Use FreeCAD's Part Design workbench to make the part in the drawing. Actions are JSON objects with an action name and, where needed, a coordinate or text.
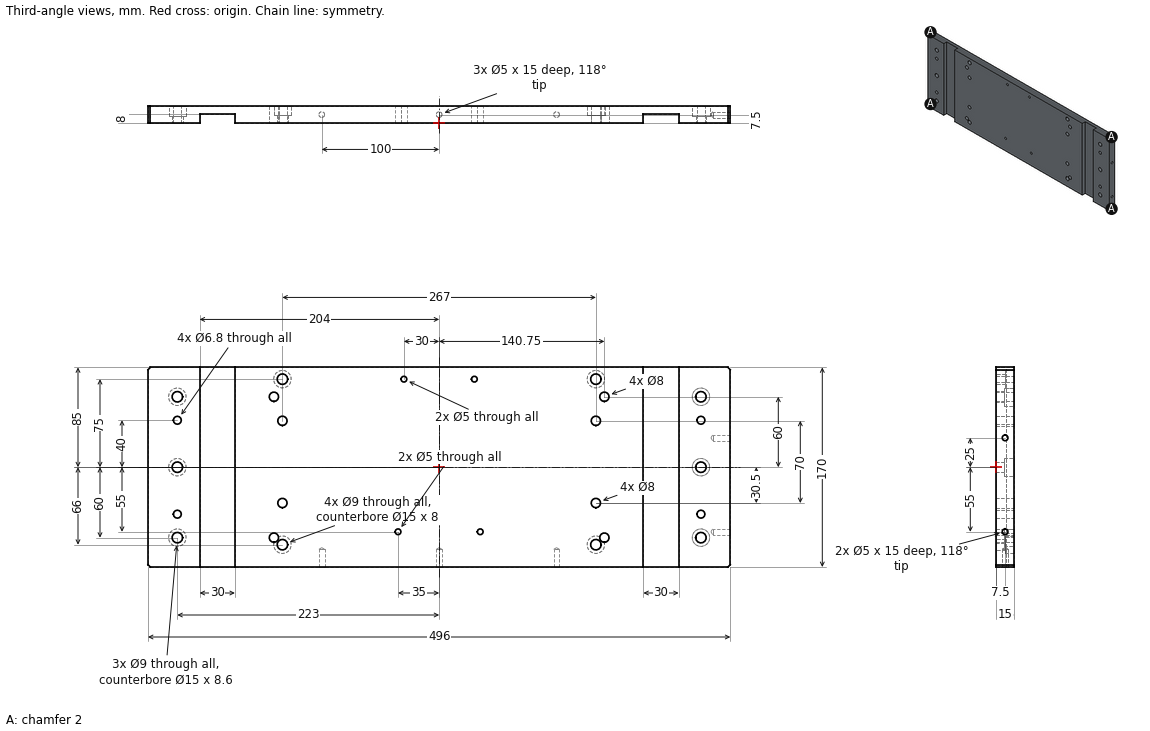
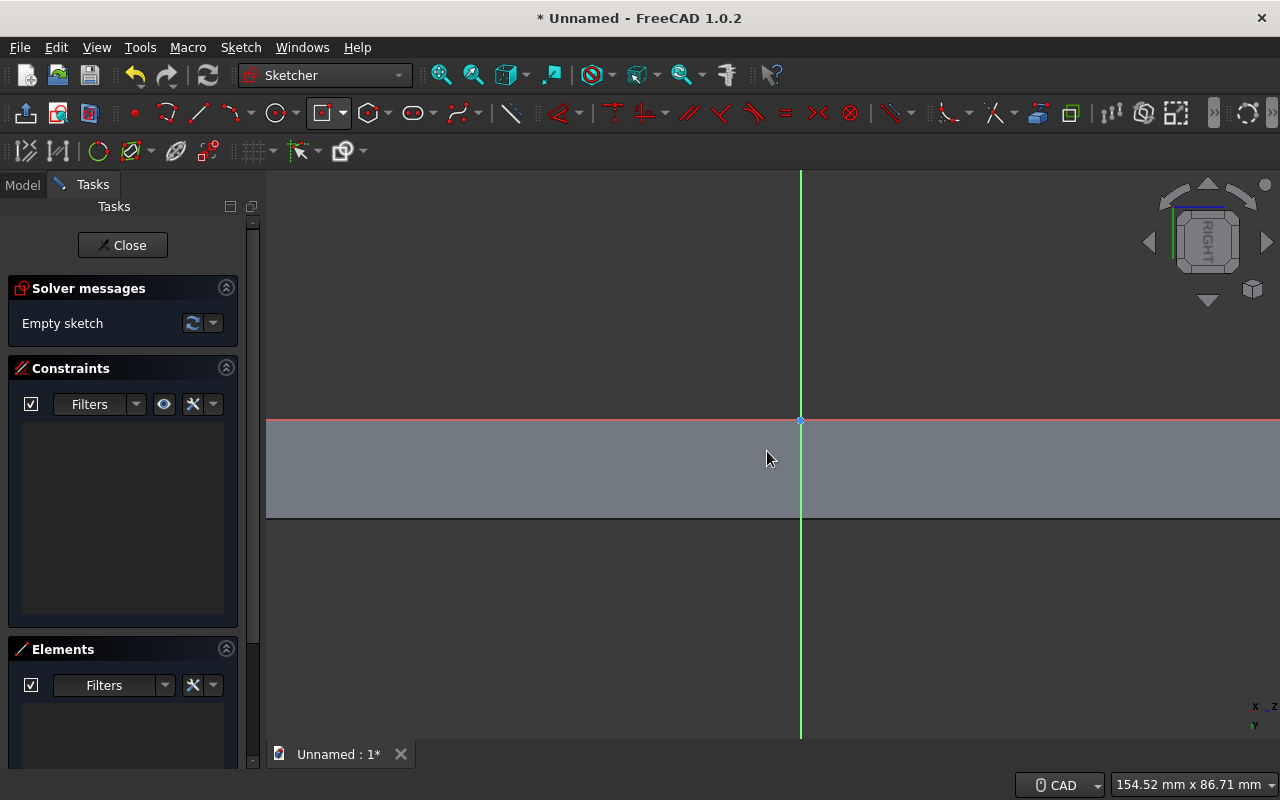
{"action": "left_click", "coordinate": [276, 114]}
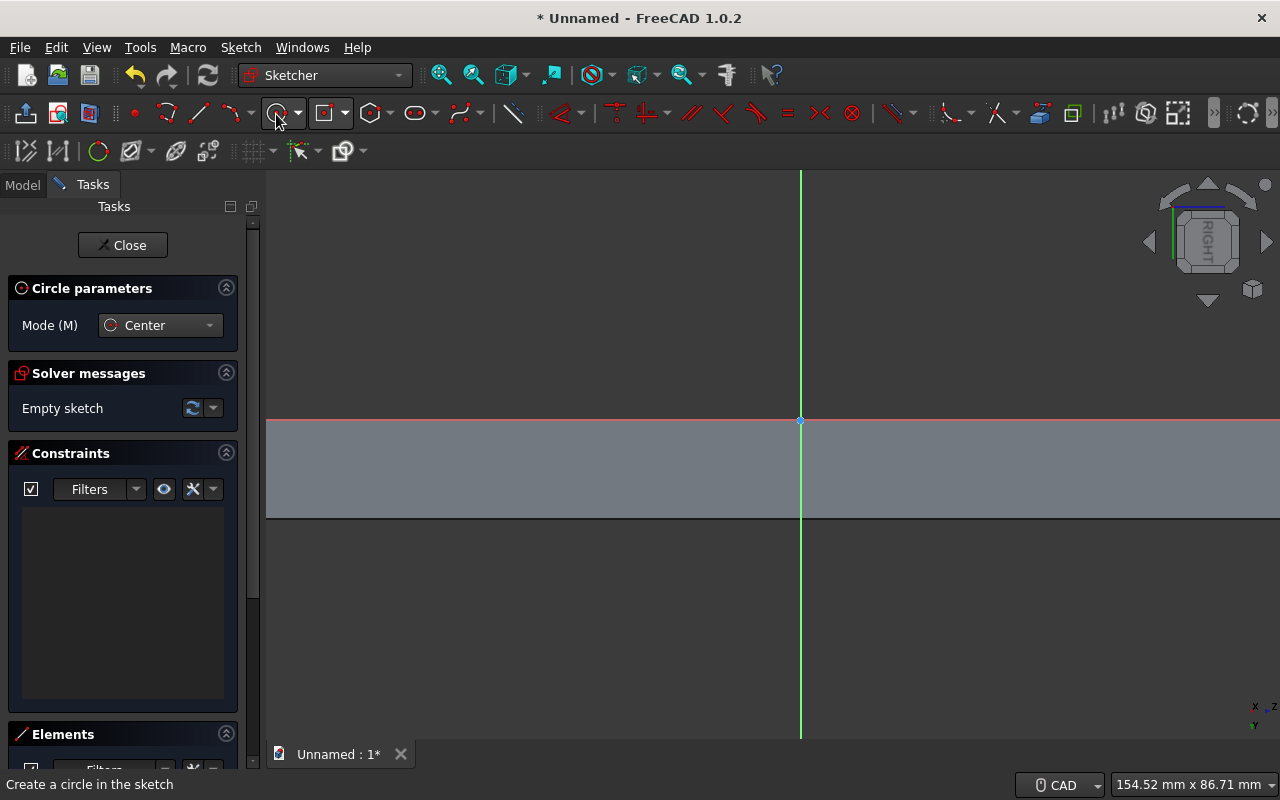
{"action": "scroll", "coordinate": [440, 470], "scroll_direction": "up", "scroll_amount": 2}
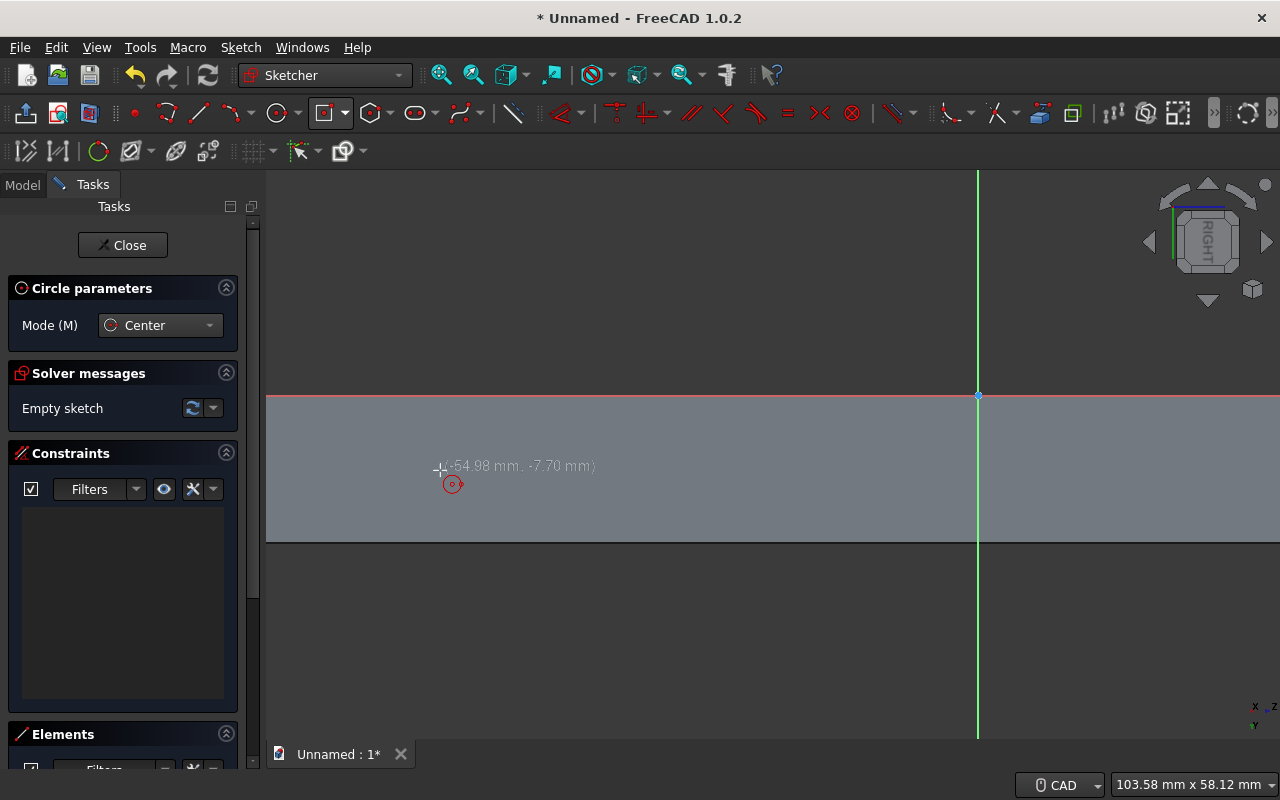
{"action": "left_click", "coordinate": [440, 469]}
{"action": "mouse_move", "coordinate": [457, 452]}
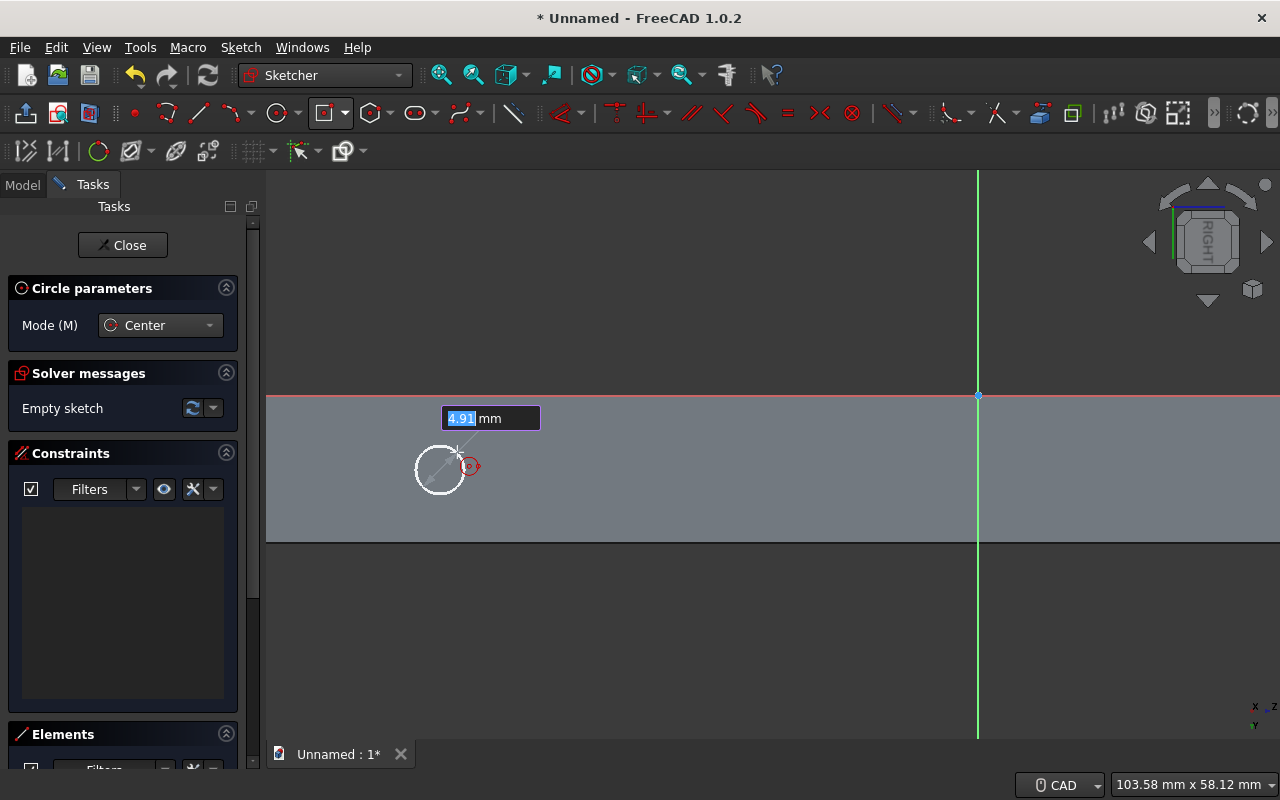
{"action": "type", "text": "5"}
{"action": "key", "text": "Return"}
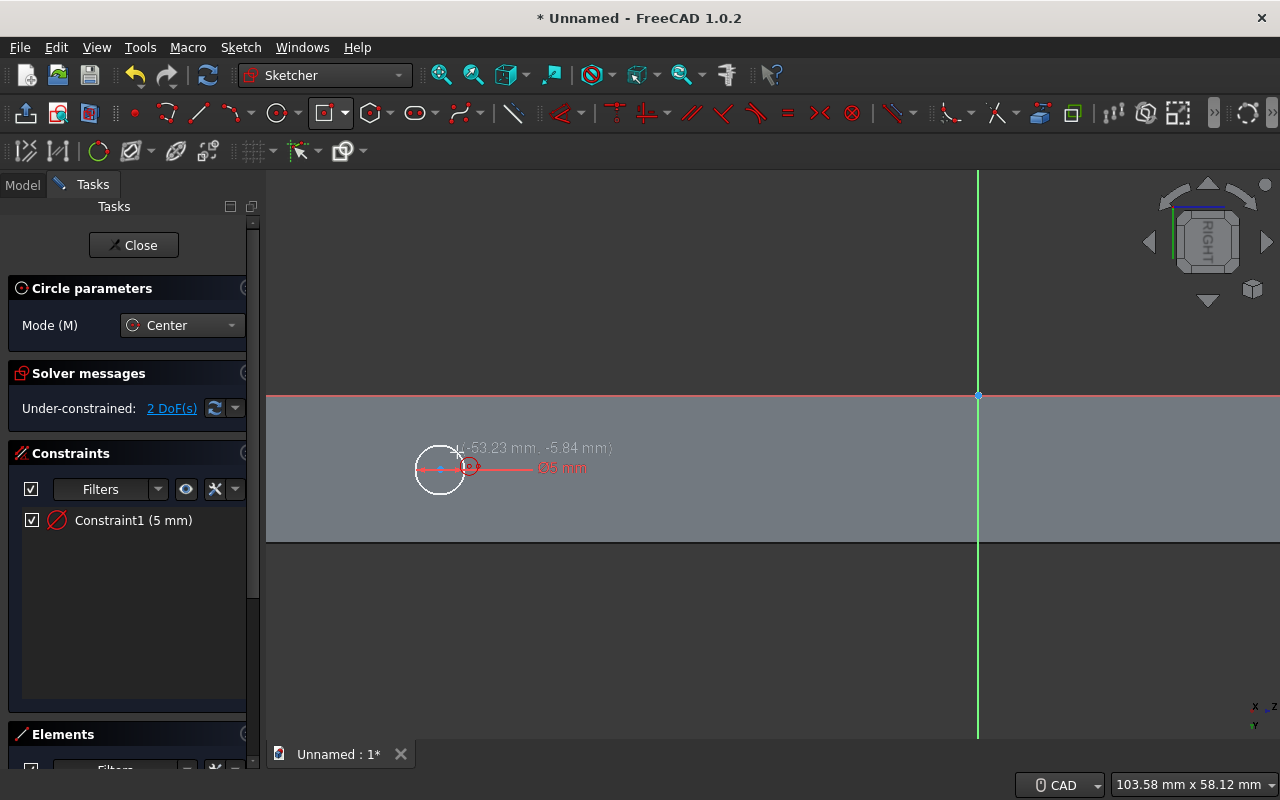
{"action": "scroll", "coordinate": [447, 474], "scroll_direction": "down", "scroll_amount": 2}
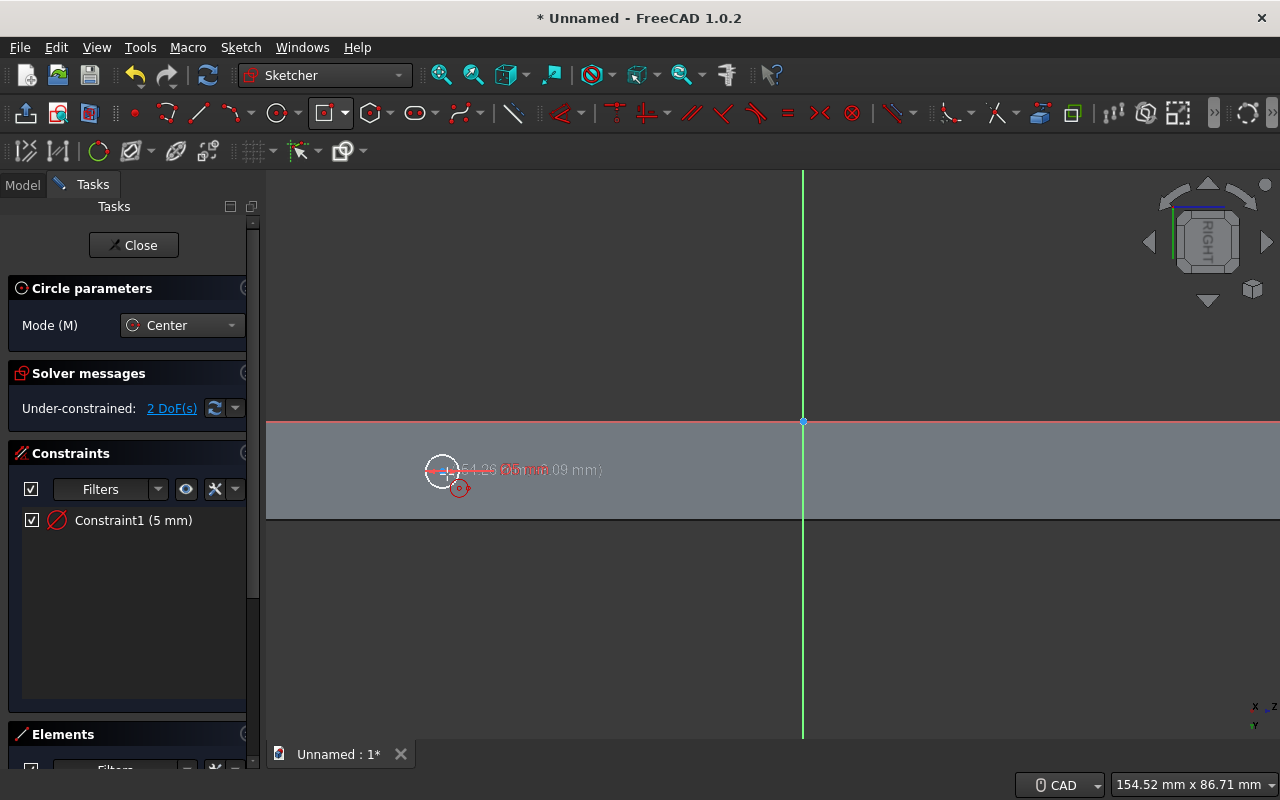
{"action": "scroll", "coordinate": [967, 471], "scroll_direction": "up", "scroll_amount": 2}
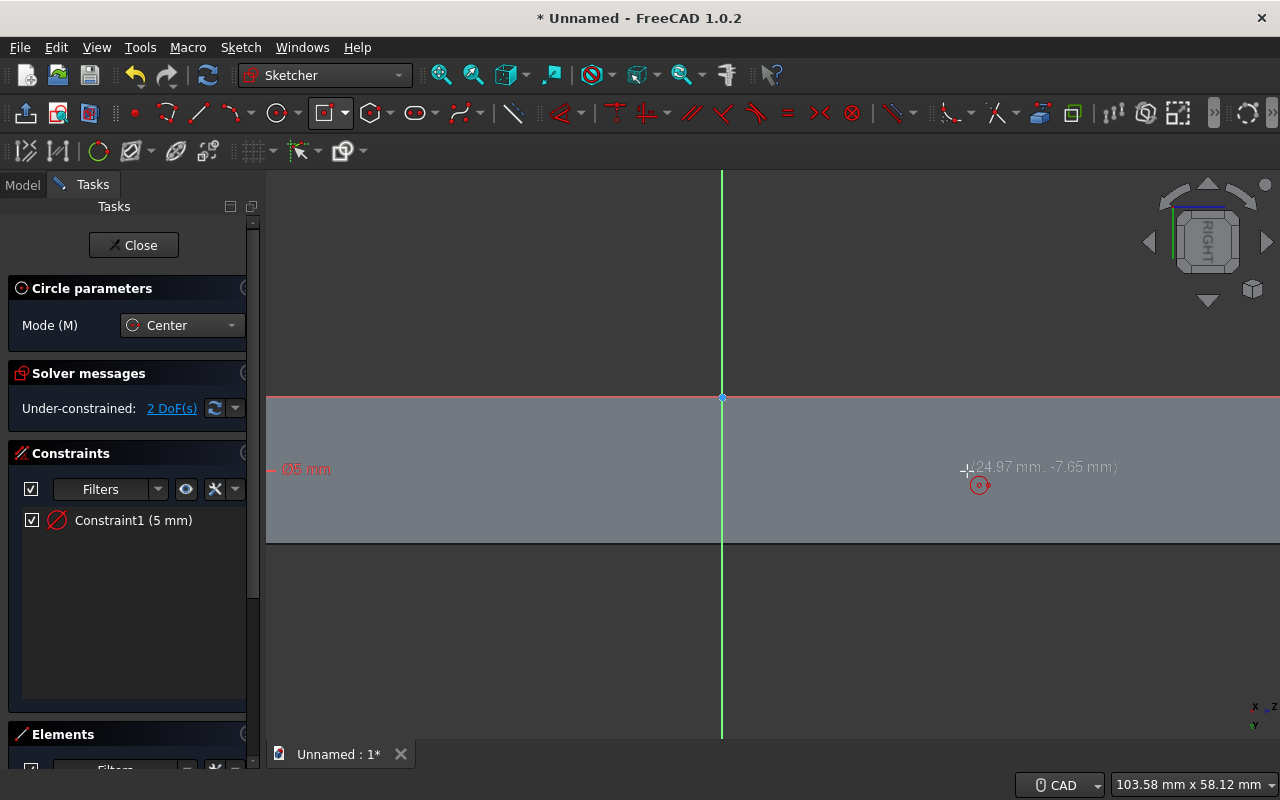
{"action": "left_click", "coordinate": [967, 471]}
{"action": "mouse_move", "coordinate": [984, 453]}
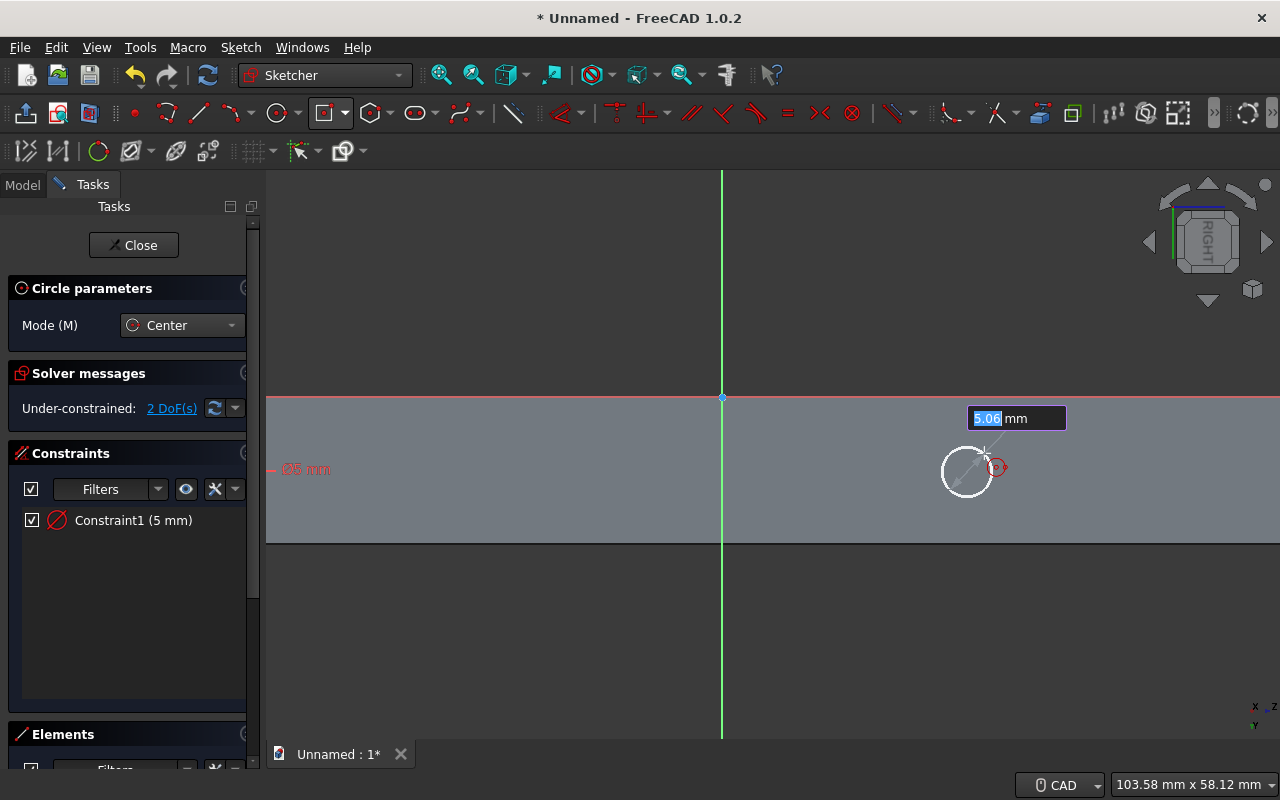
{"action": "type", "text": "5"}
{"action": "key", "text": "Return"}
{"action": "key", "text": "Escape"}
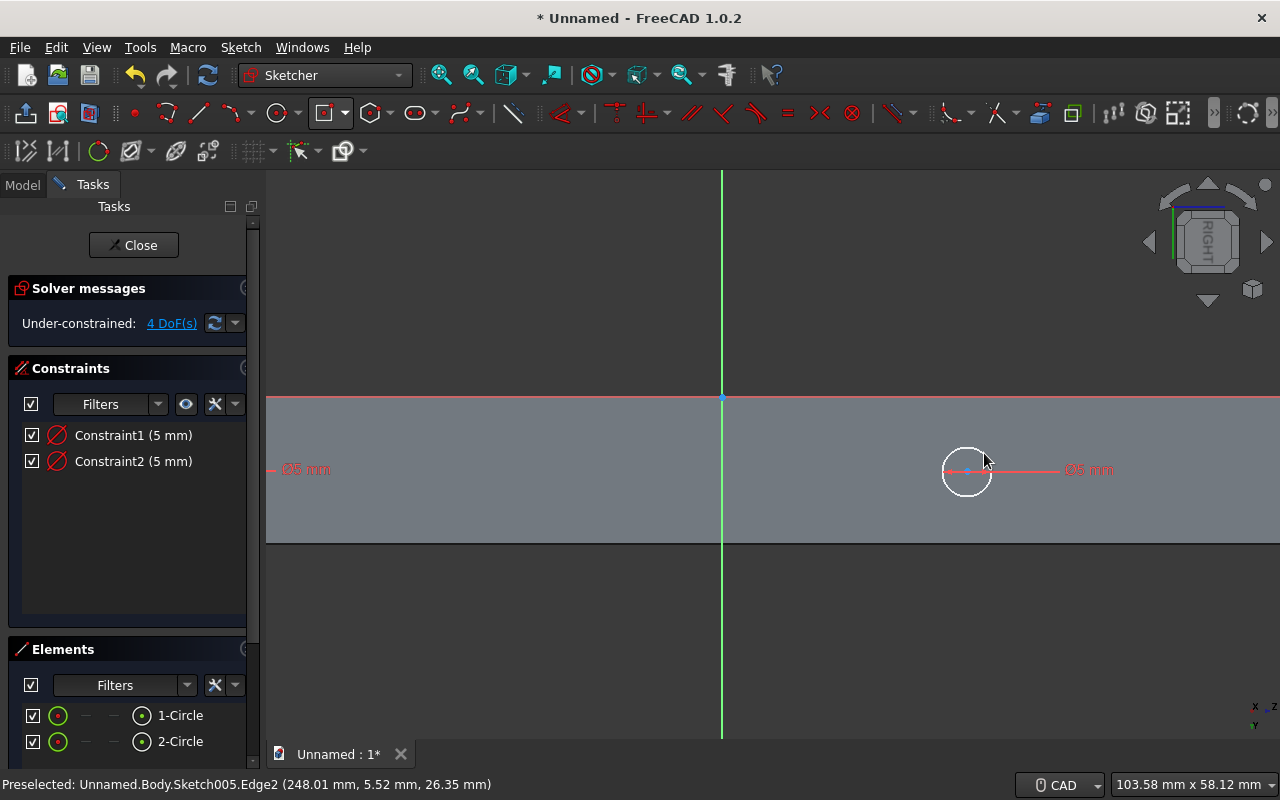
{"action": "left_click", "coordinate": [560, 114]}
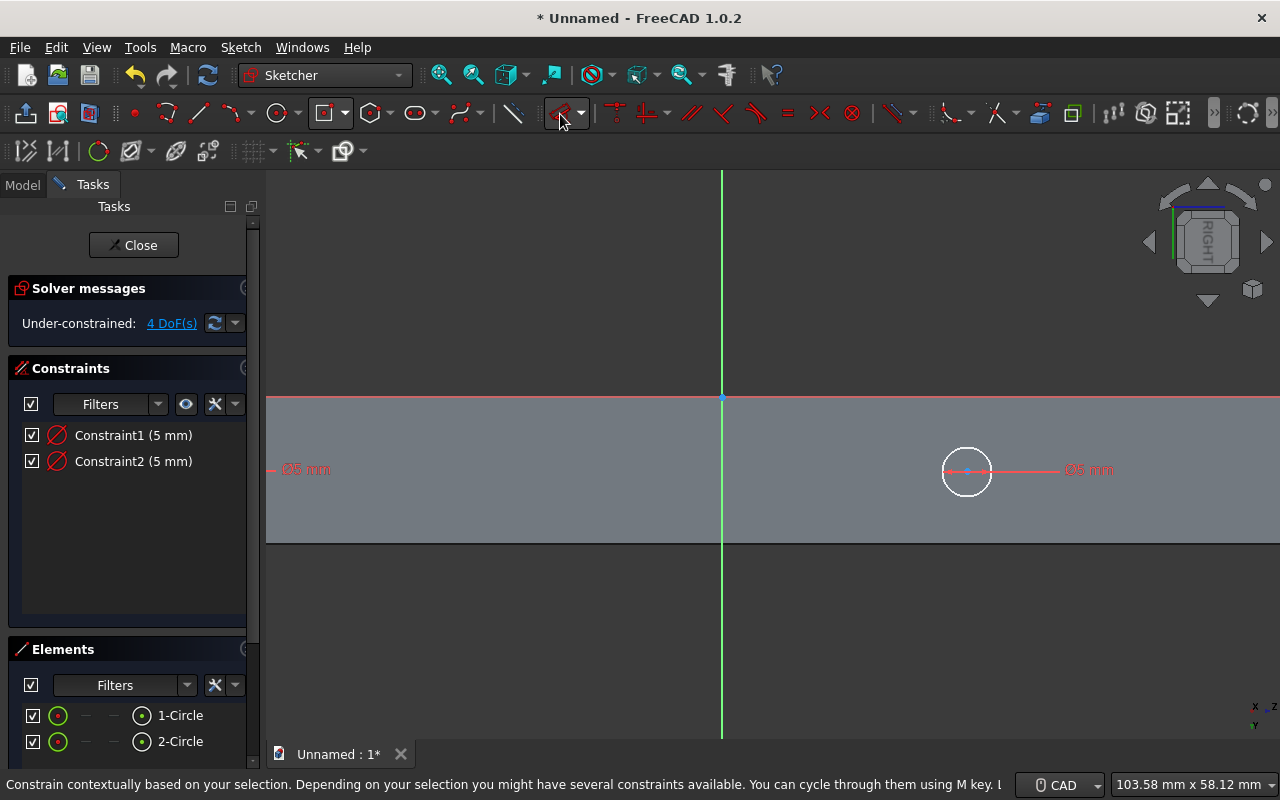
{"action": "scroll", "coordinate": [967, 471], "scroll_direction": "down", "scroll_amount": 2}